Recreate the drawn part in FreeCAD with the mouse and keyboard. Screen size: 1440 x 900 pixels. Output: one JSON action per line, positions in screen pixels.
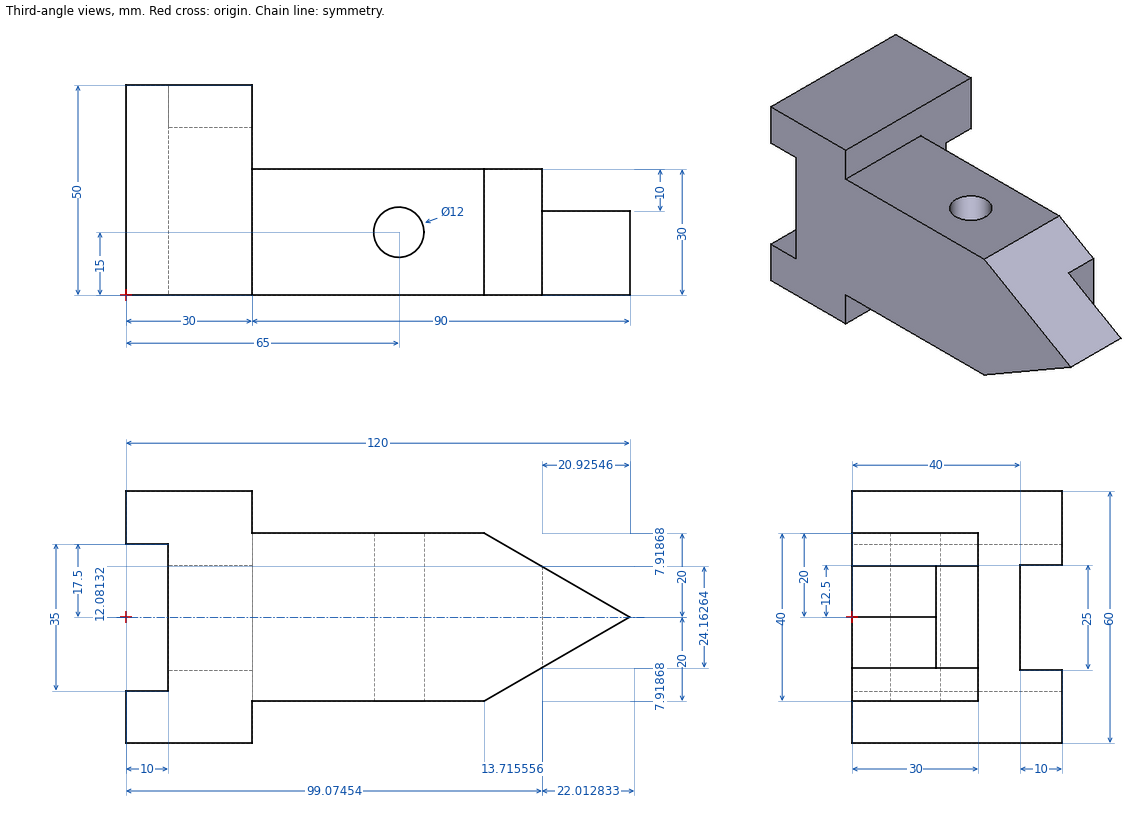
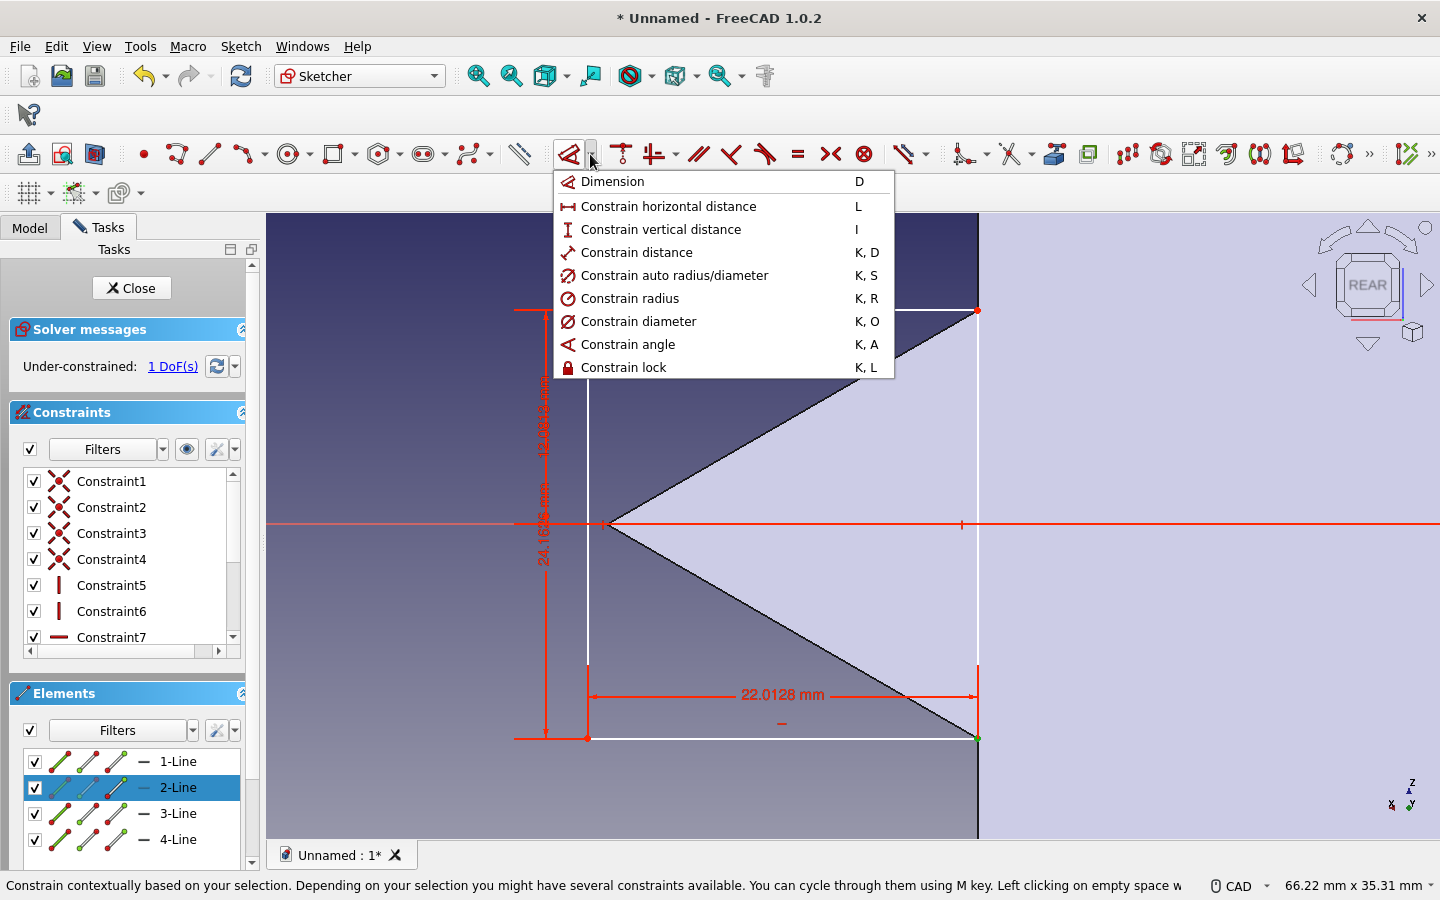
{"action": "left_click", "coordinate": [724, 206]}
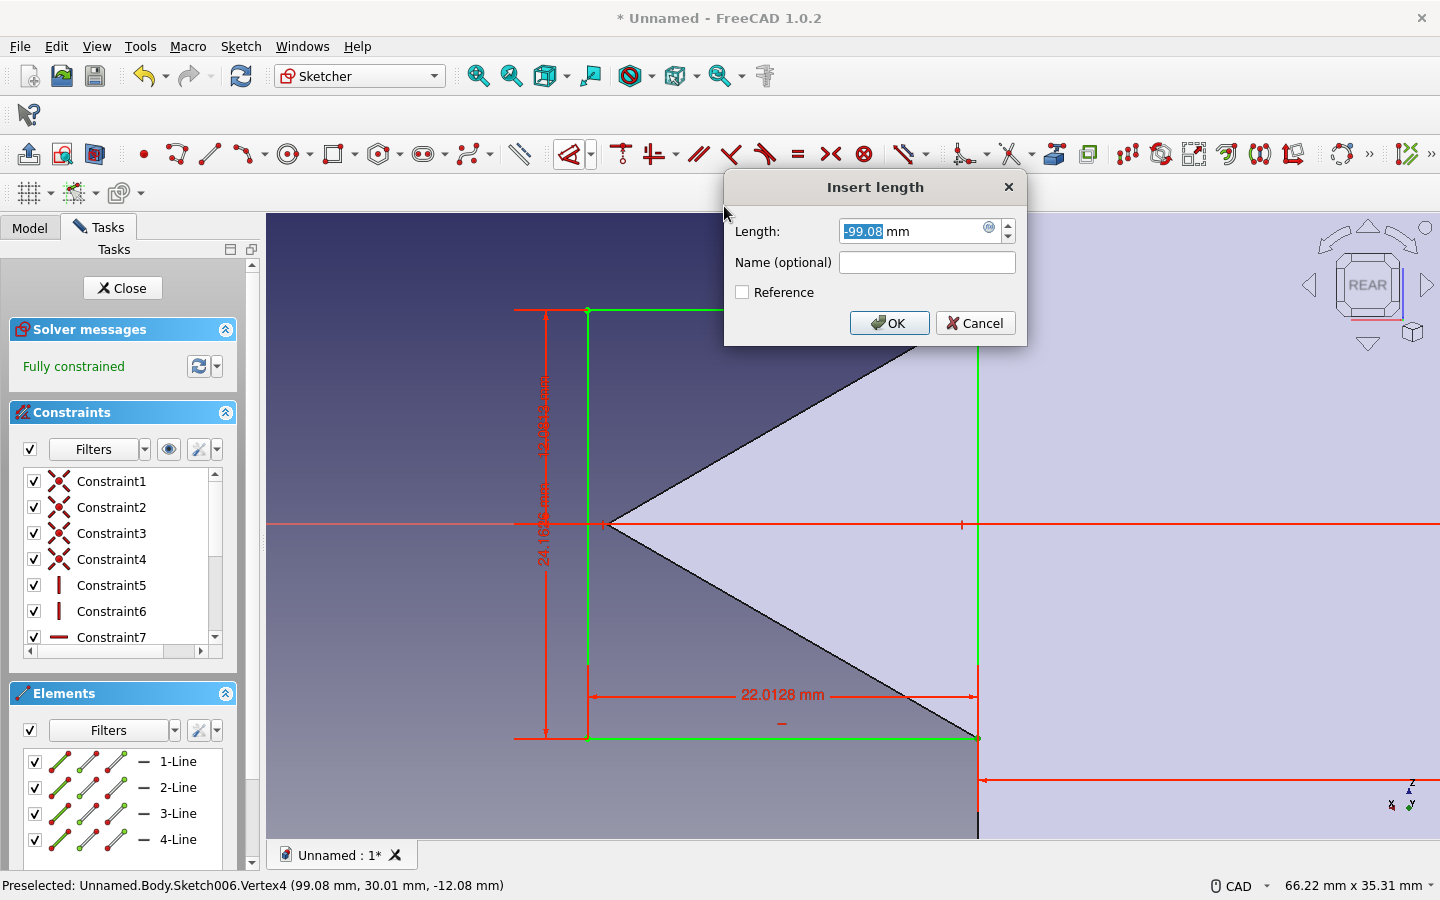
{"action": "type", "text": "-99.07454"}
{"action": "key", "text": "Return"}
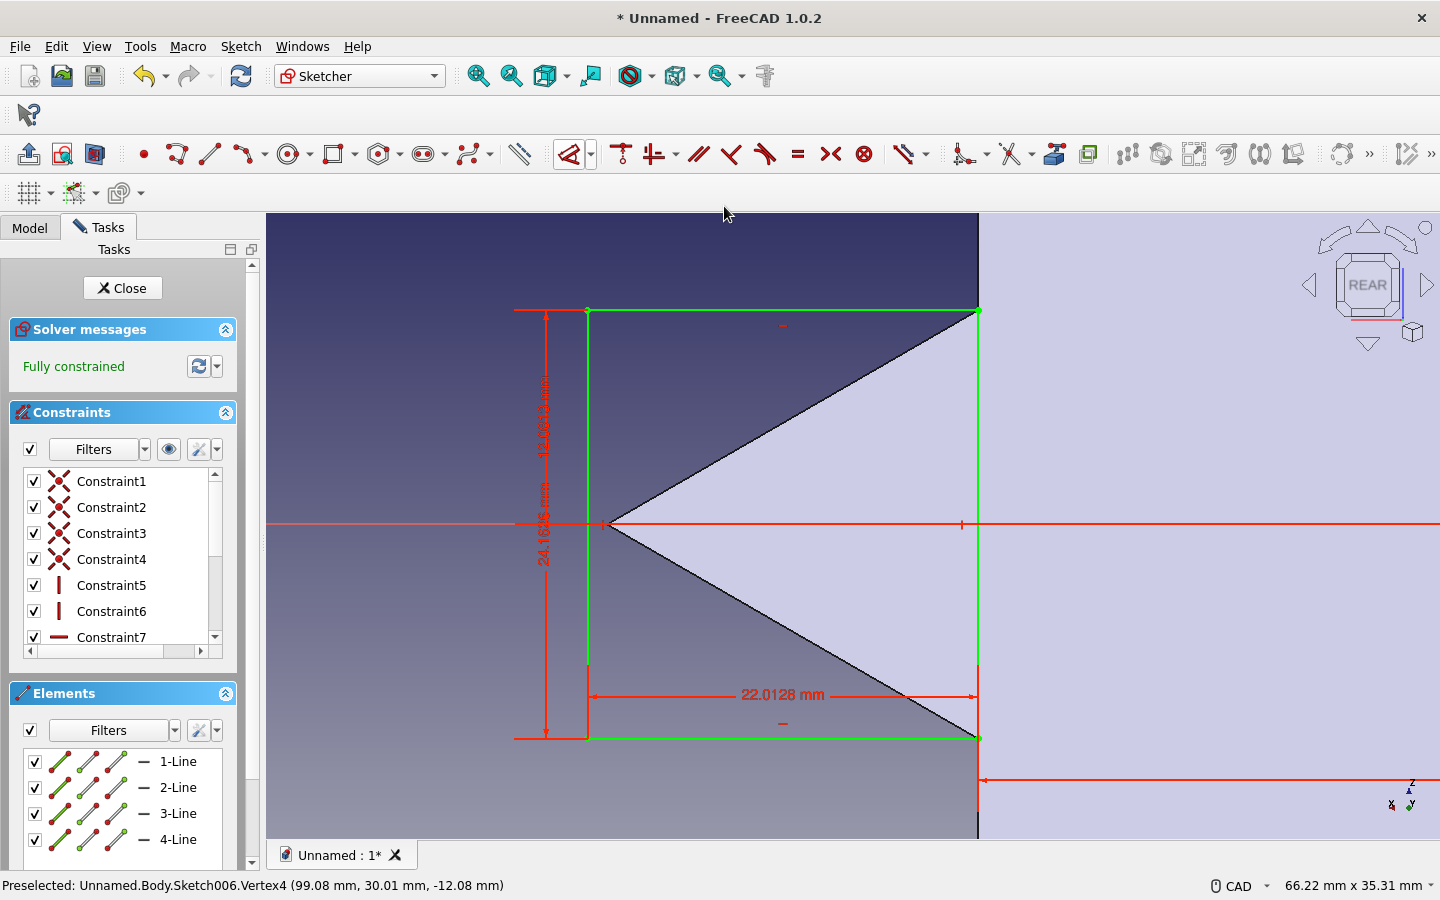
{"action": "left_click", "coordinate": [123, 288]}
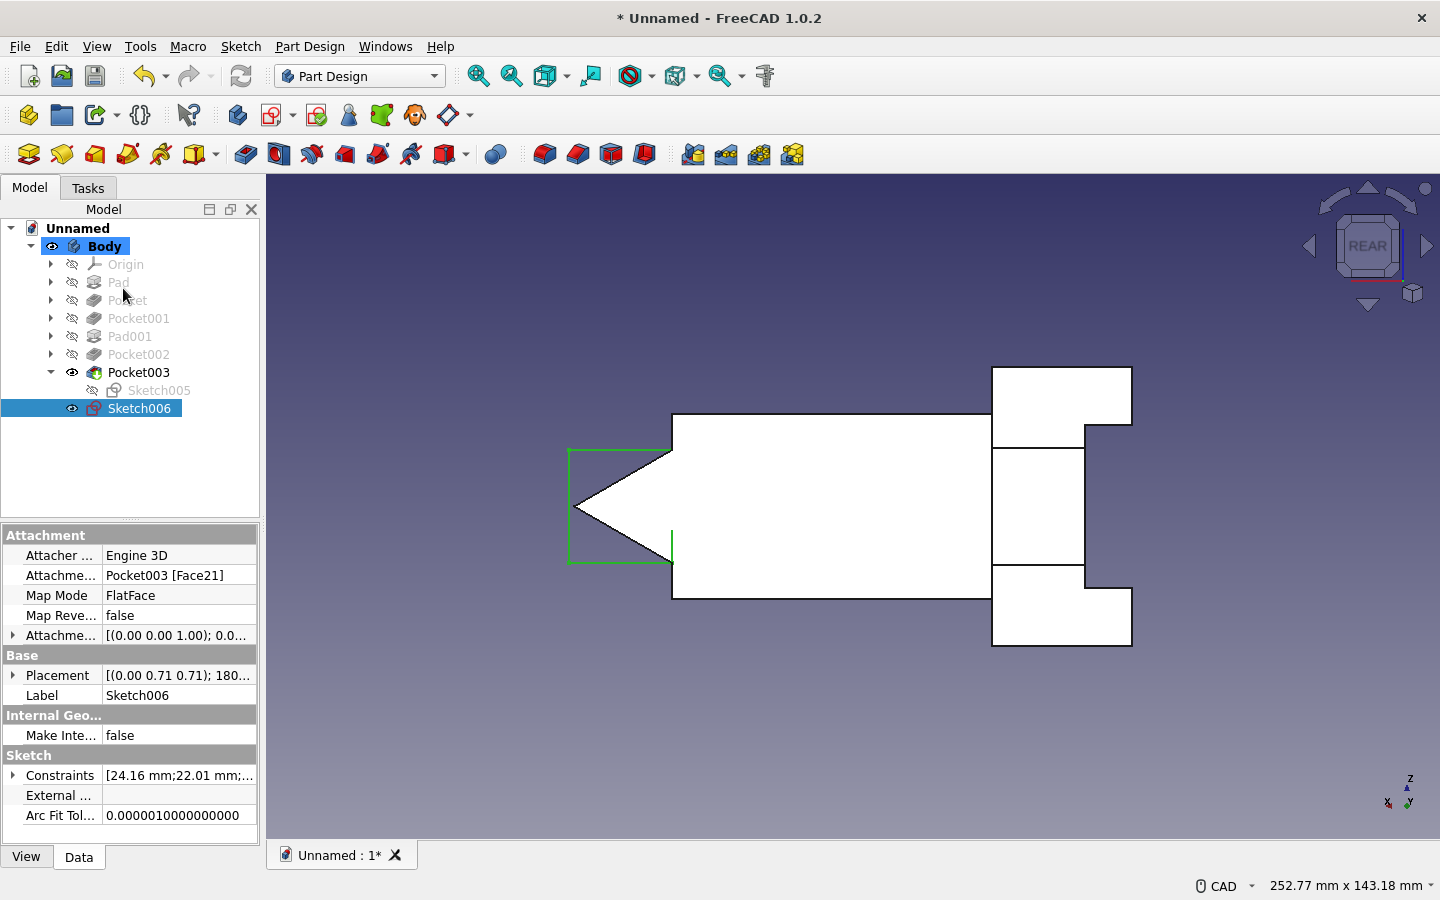
{"action": "left_click", "coordinate": [246, 154]}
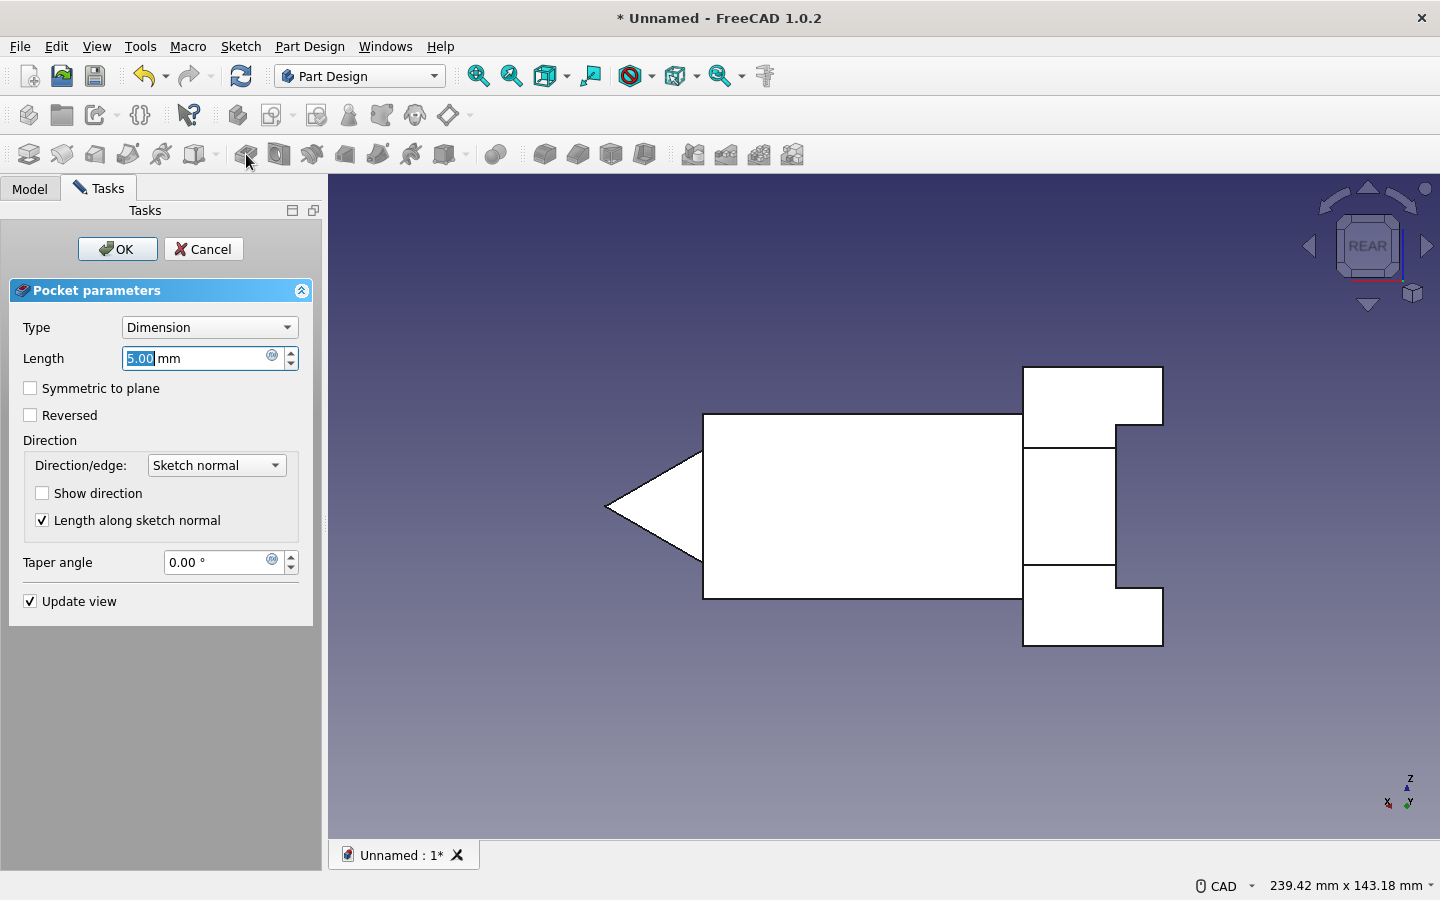
{"action": "type", "text": "10"}
{"action": "key", "text": "Tab"}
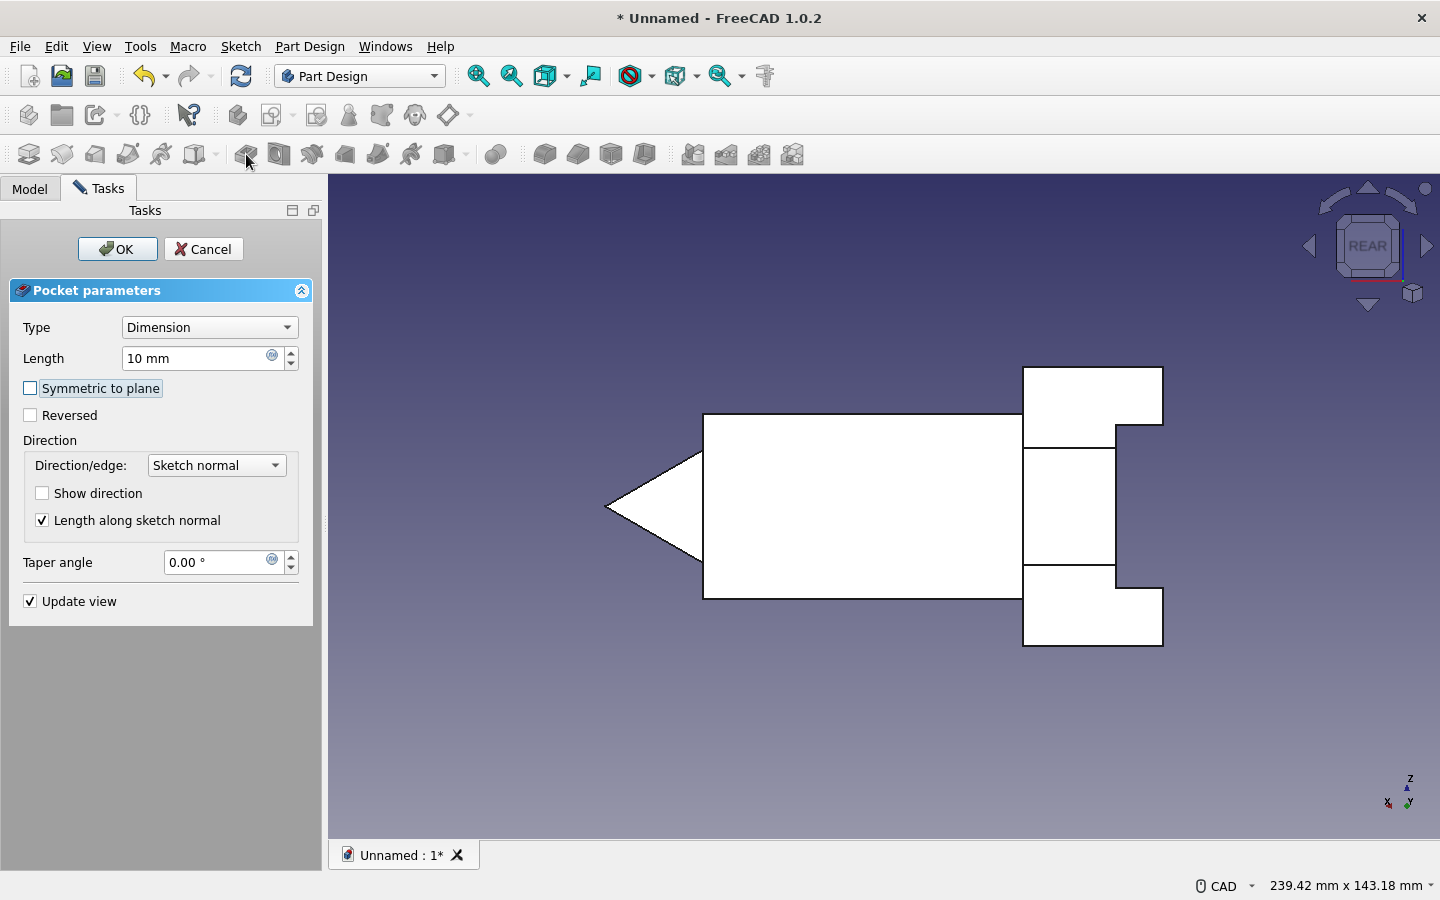
{"action": "left_click", "coordinate": [118, 249]}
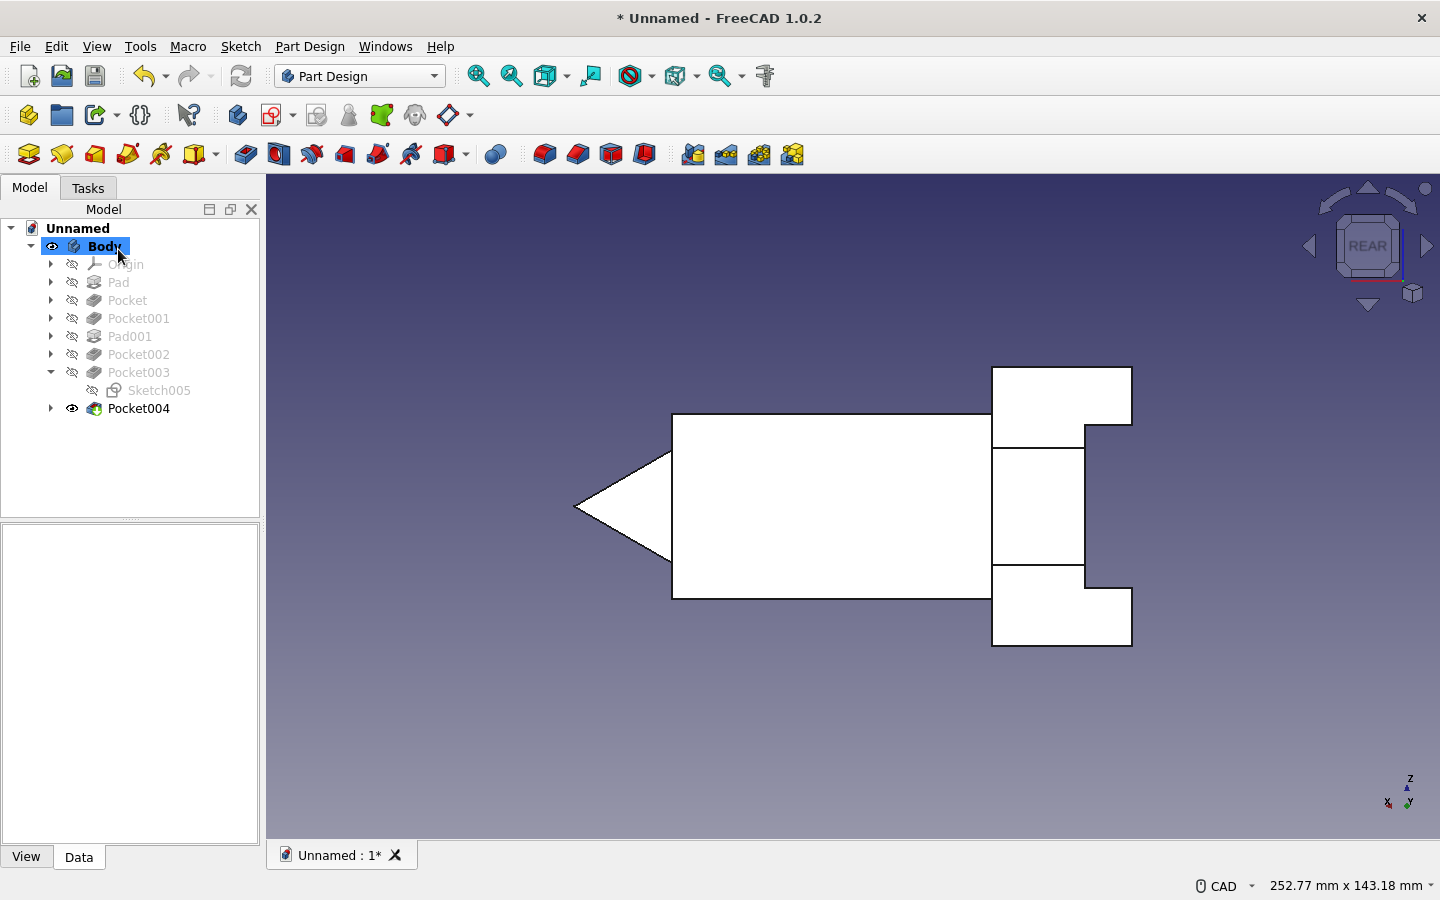
{"action": "left_click", "coordinate": [786, 506]}